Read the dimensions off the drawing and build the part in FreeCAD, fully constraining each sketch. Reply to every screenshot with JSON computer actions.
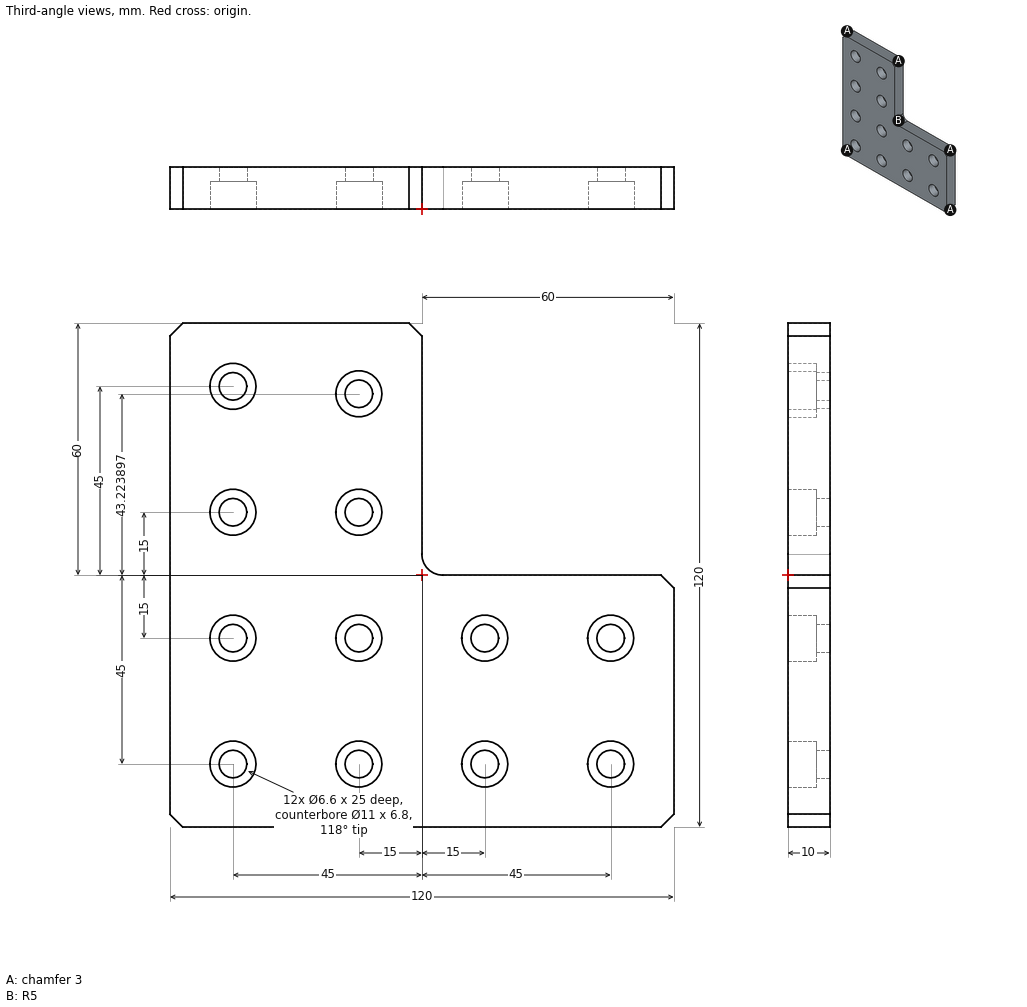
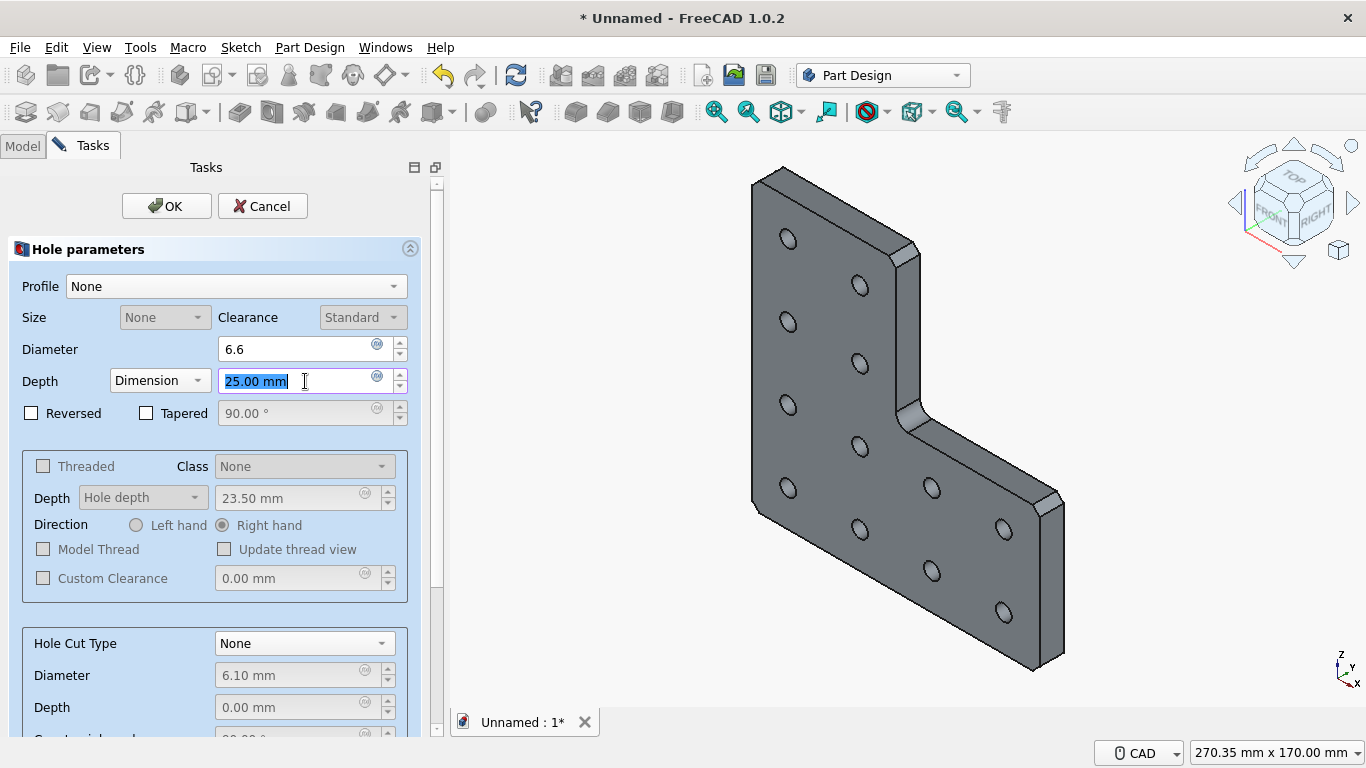
{"action": "type", "text": "25"}
{"action": "key", "text": "Tab"}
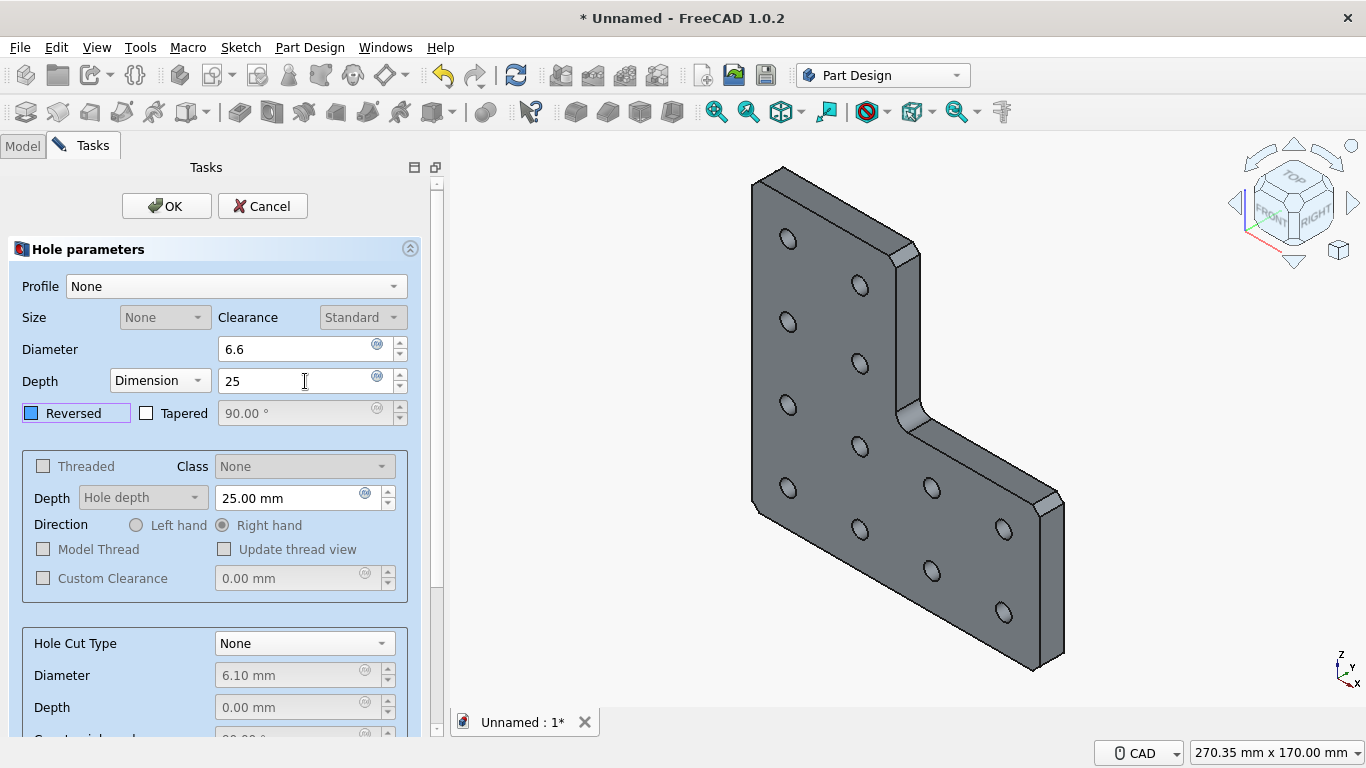
{"action": "left_click", "coordinate": [306, 644]}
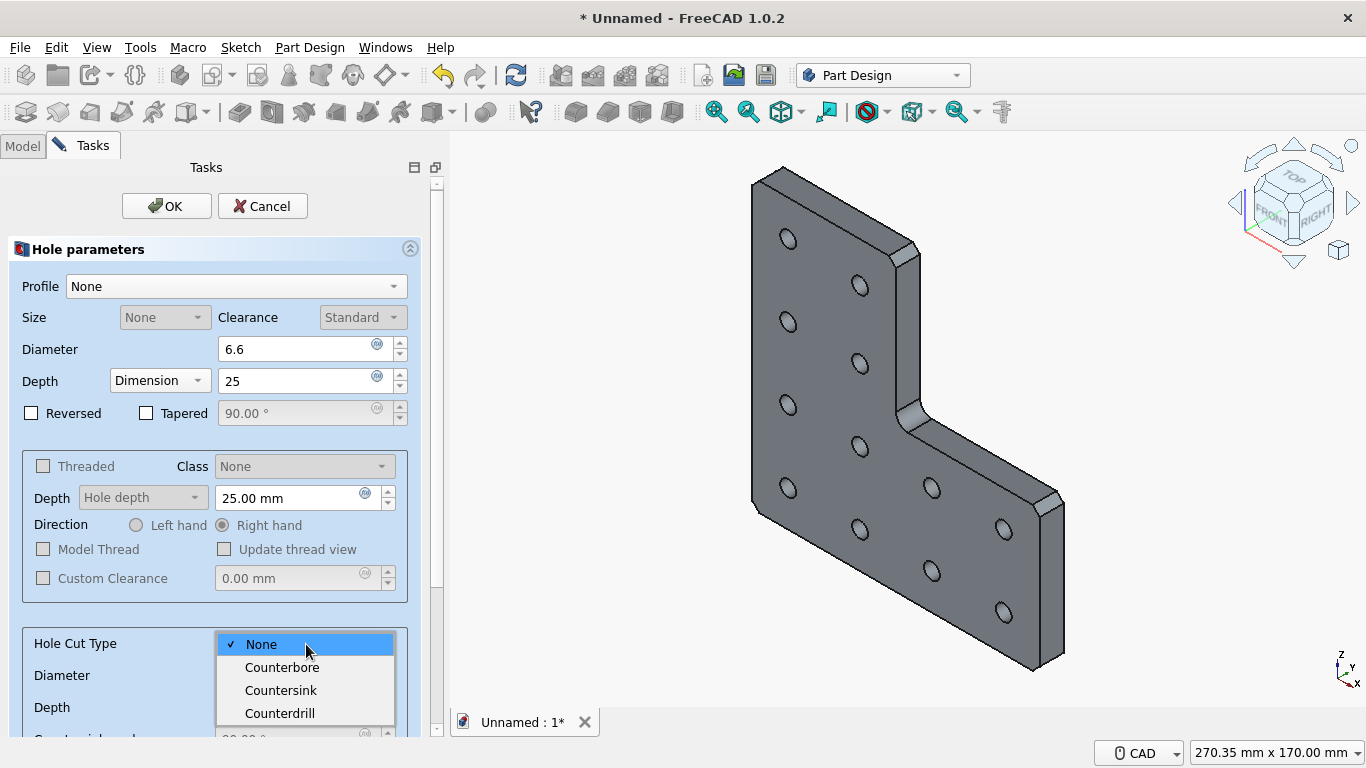
{"action": "left_click", "coordinate": [304, 668]}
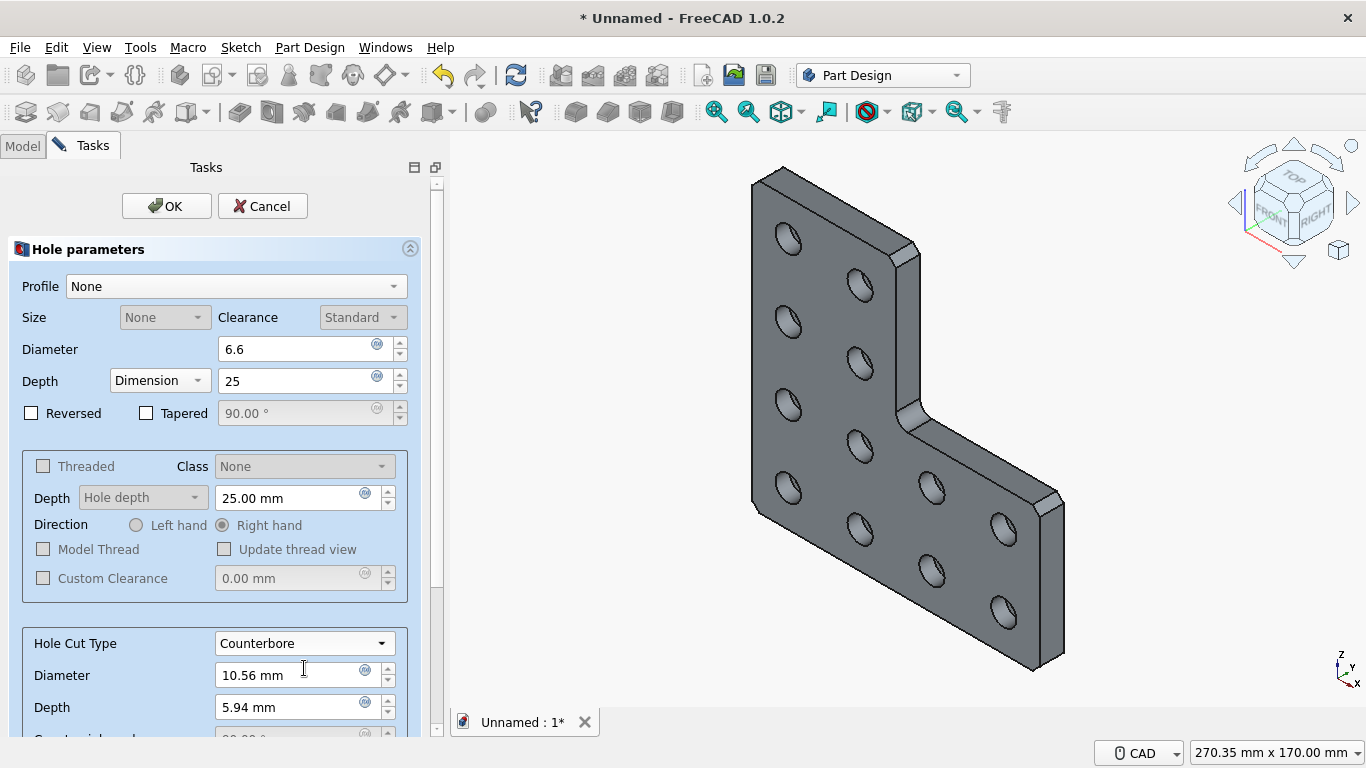
{"action": "triple_click", "coordinate": [298, 675]}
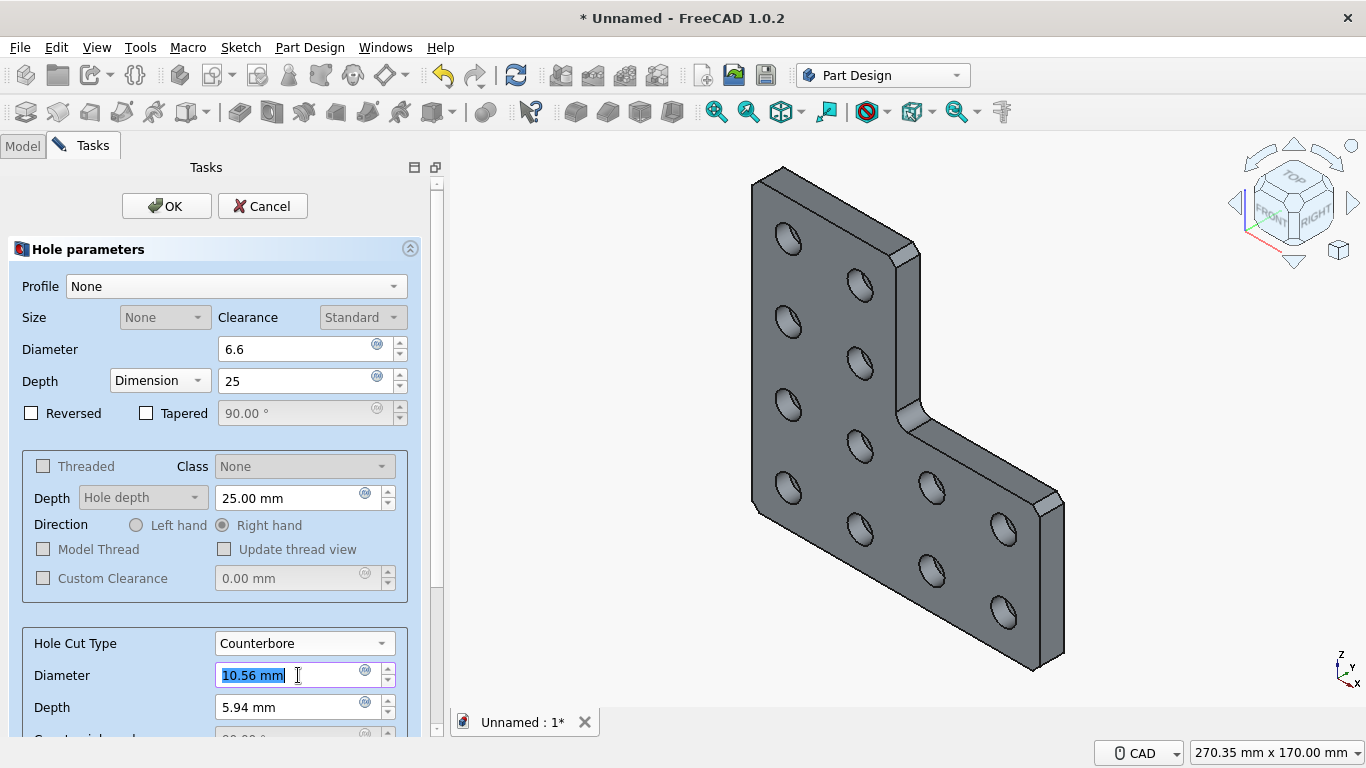
{"action": "type", "text": "11"}
{"action": "key", "text": "Tab"}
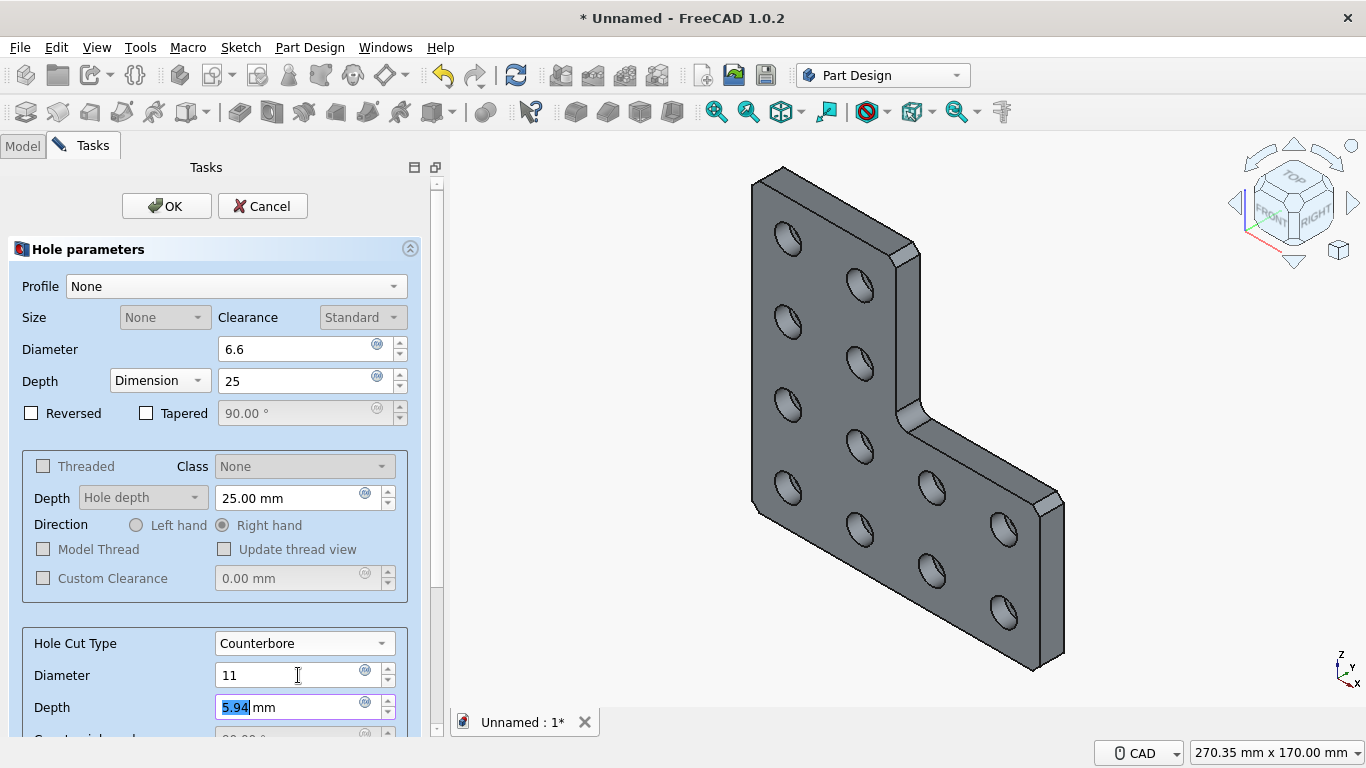
{"action": "type", "text": "6.8"}
{"action": "key", "text": "Tab"}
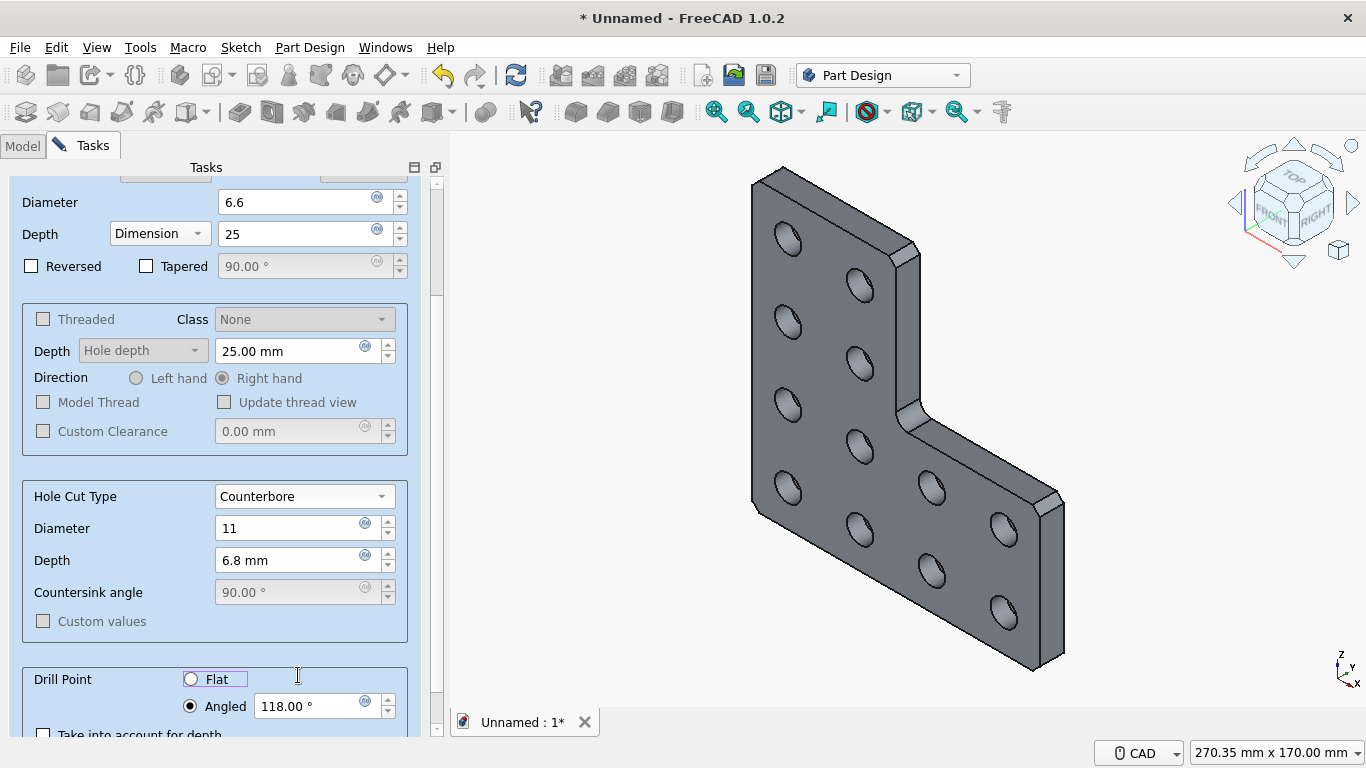
{"action": "scroll", "coordinate": [437, 456], "scroll_direction": "up", "scroll_amount": 4}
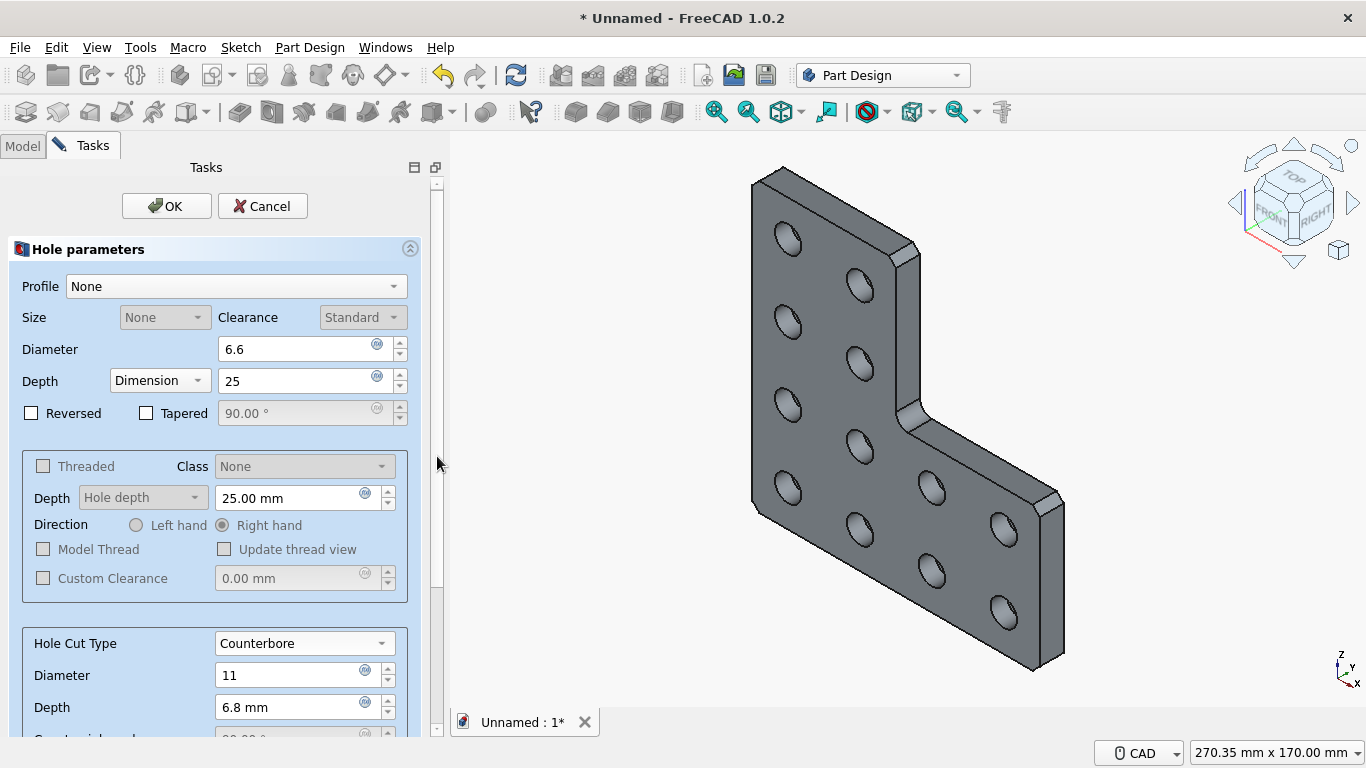
{"action": "left_click", "coordinate": [167, 206]}